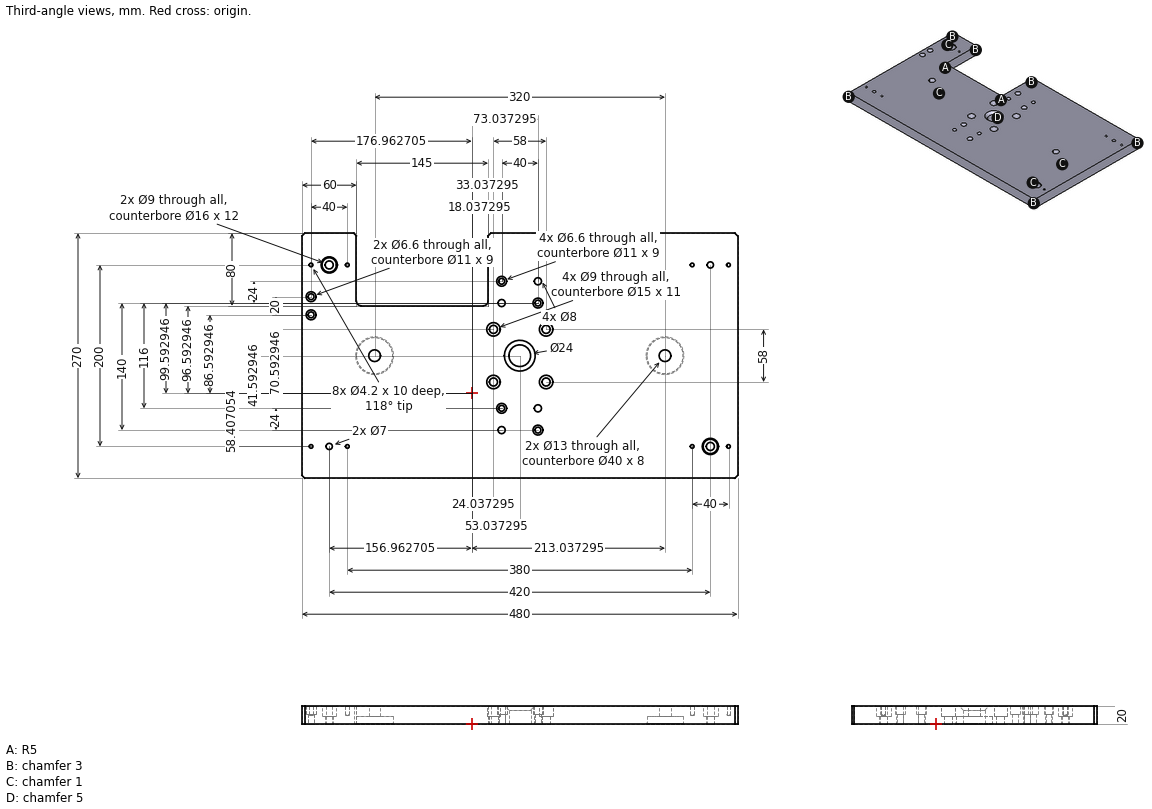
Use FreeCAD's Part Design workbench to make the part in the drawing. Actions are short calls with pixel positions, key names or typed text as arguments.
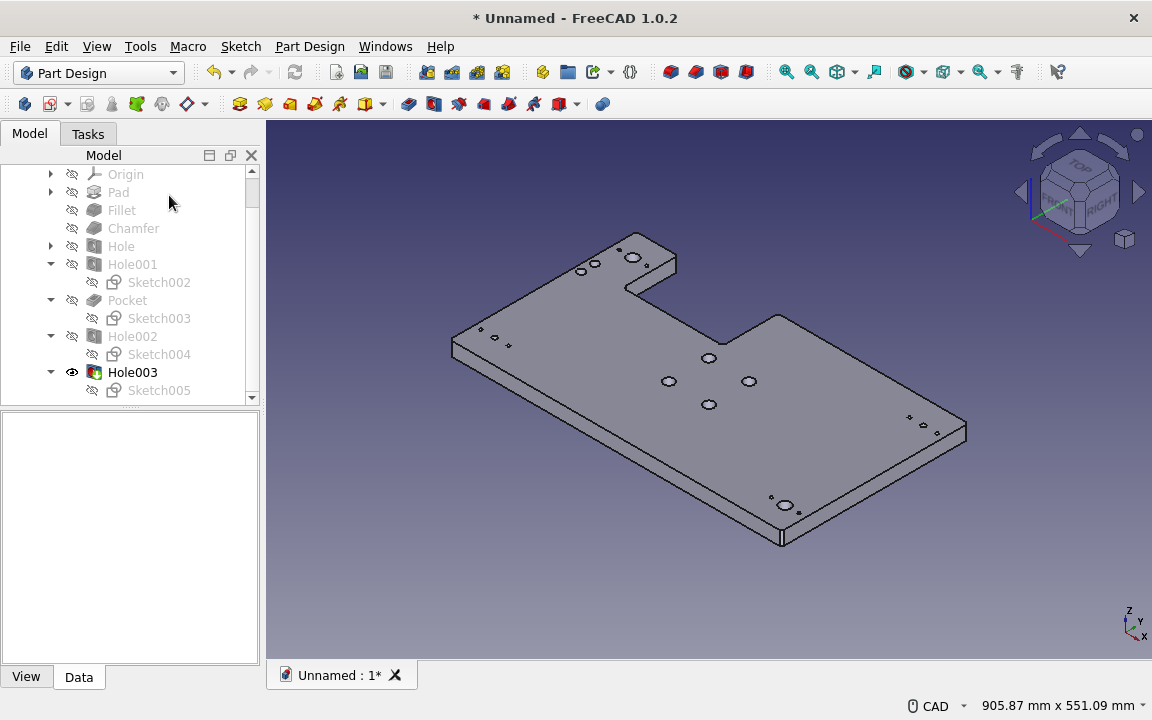
click(804, 435)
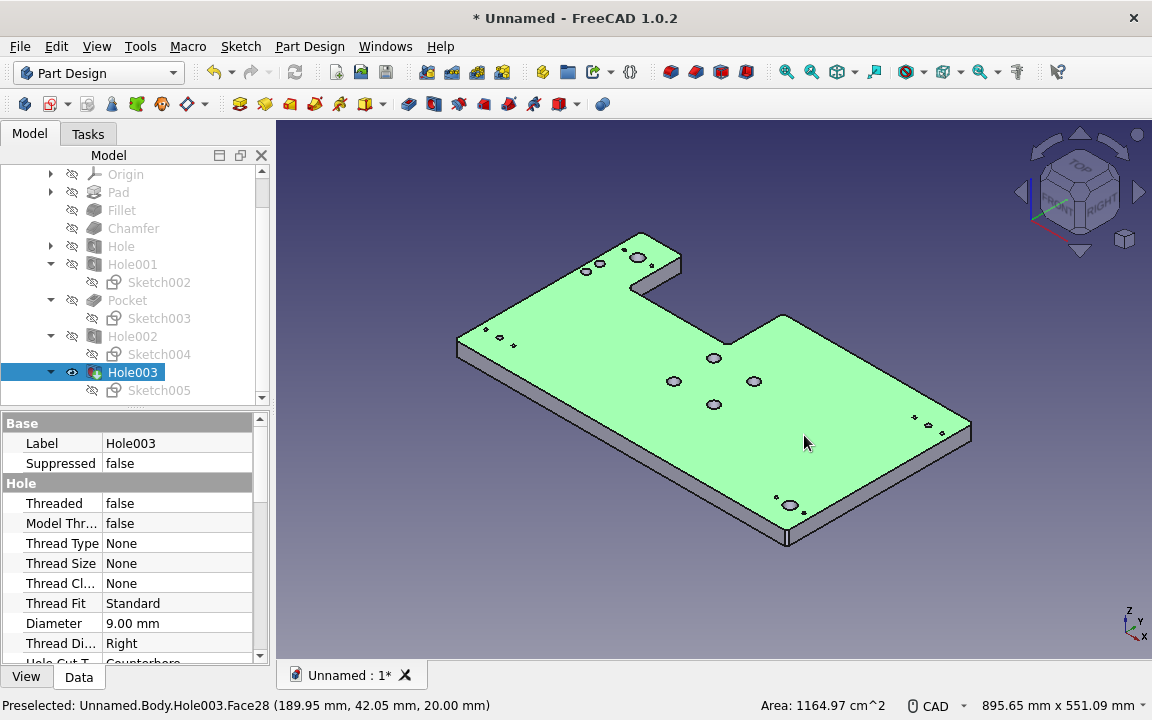
click(50, 104)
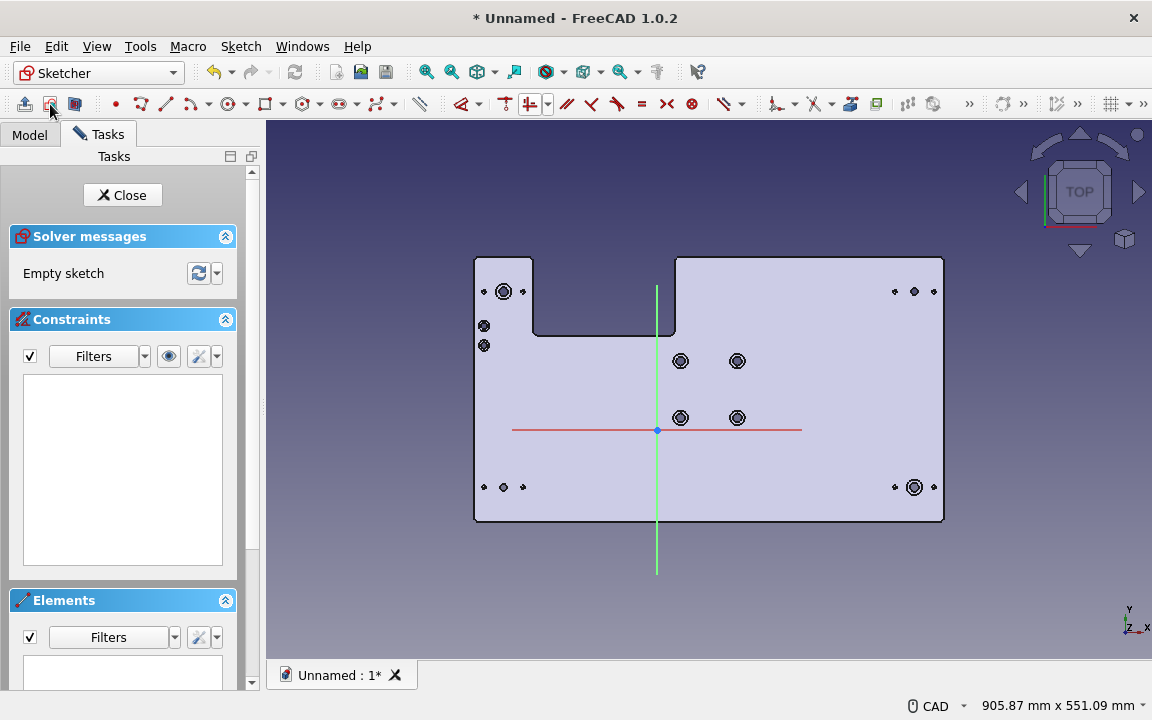
scroll(738, 390, up, 4)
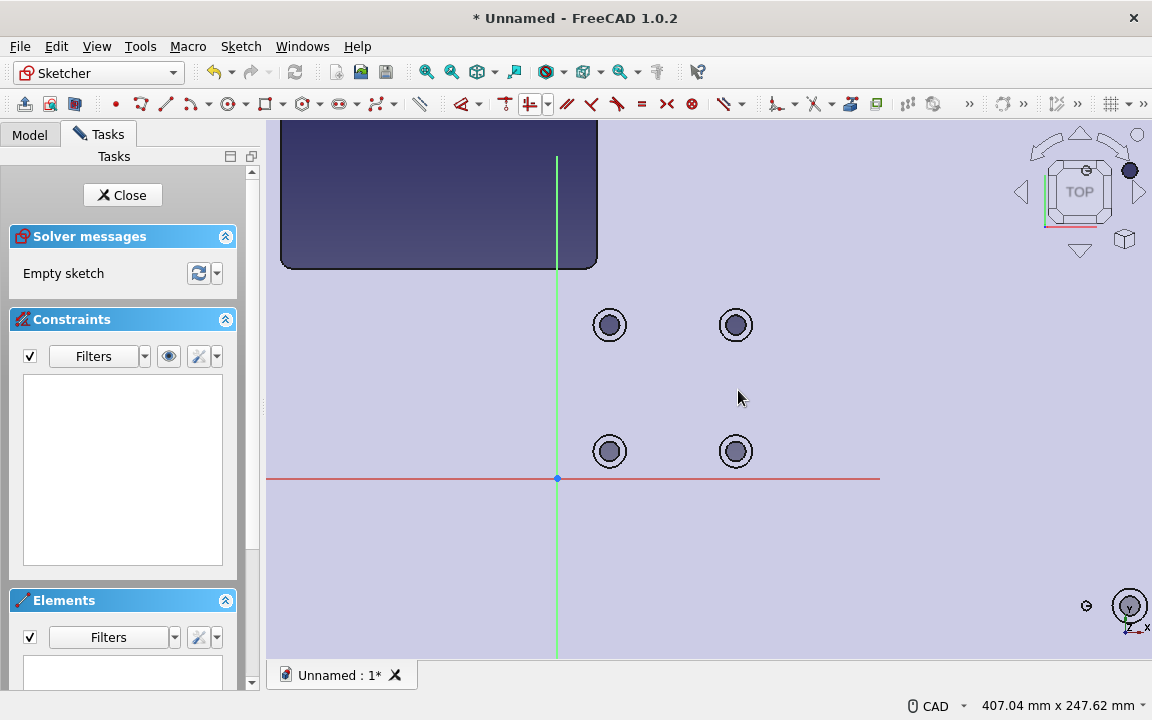
key(g)
key(c)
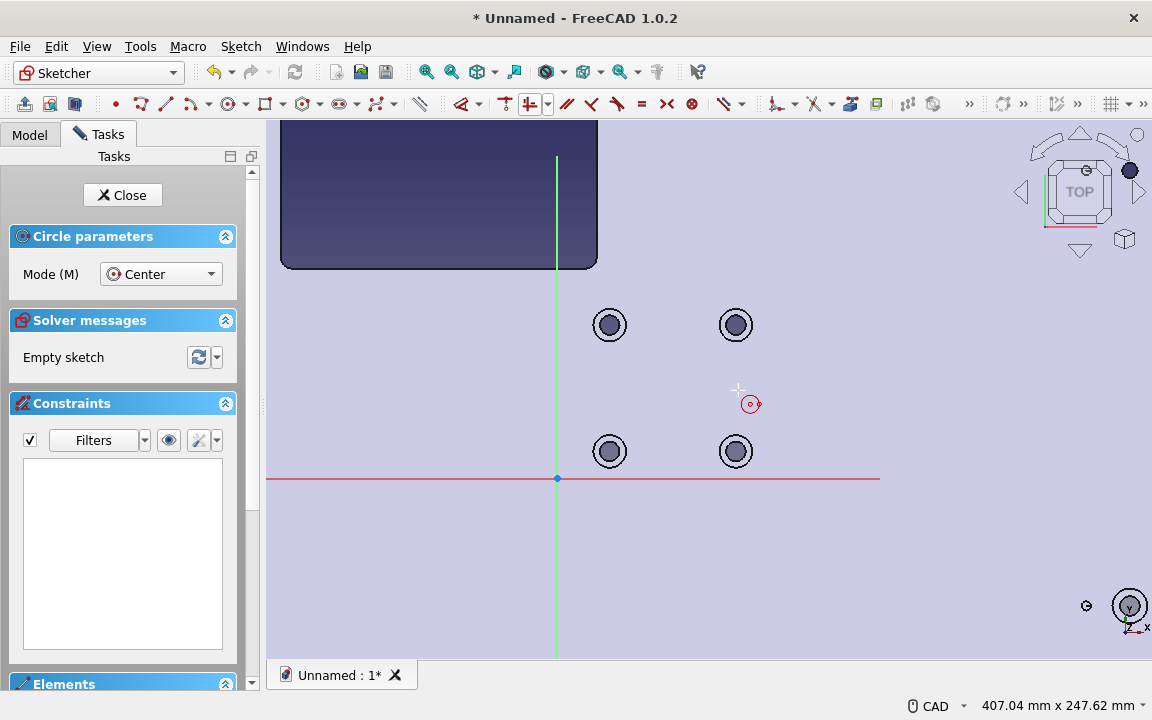
scroll(629, 210, up, 6)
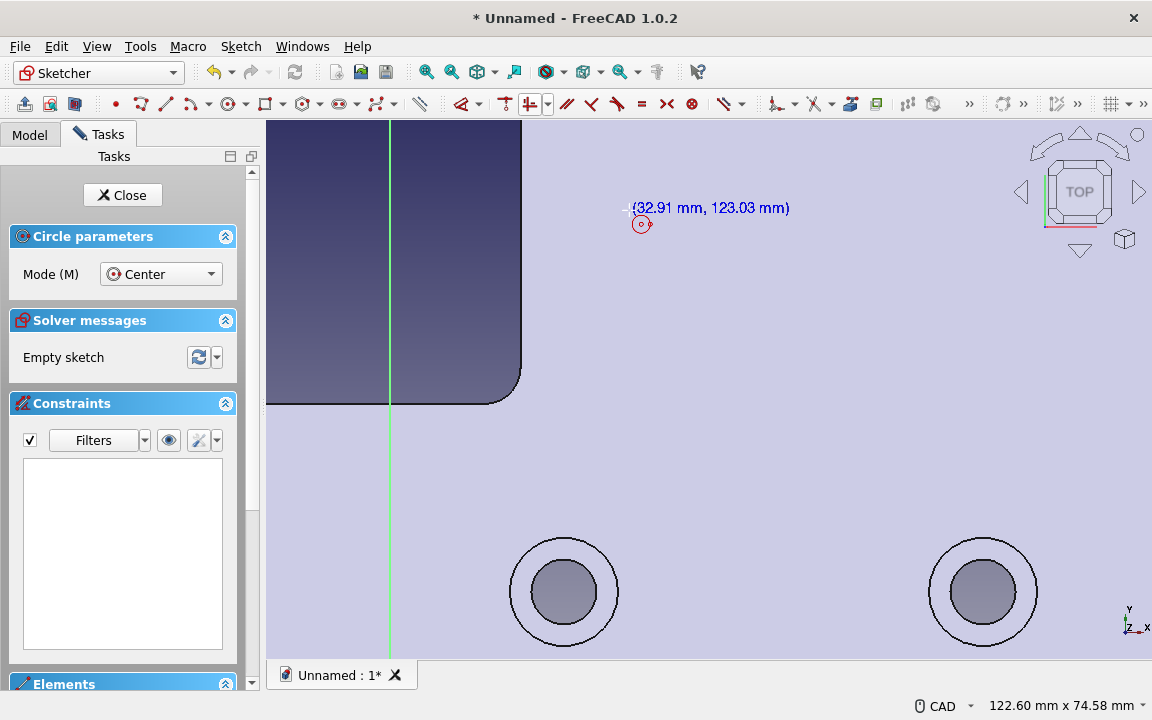
click(629, 209)
click(646, 192)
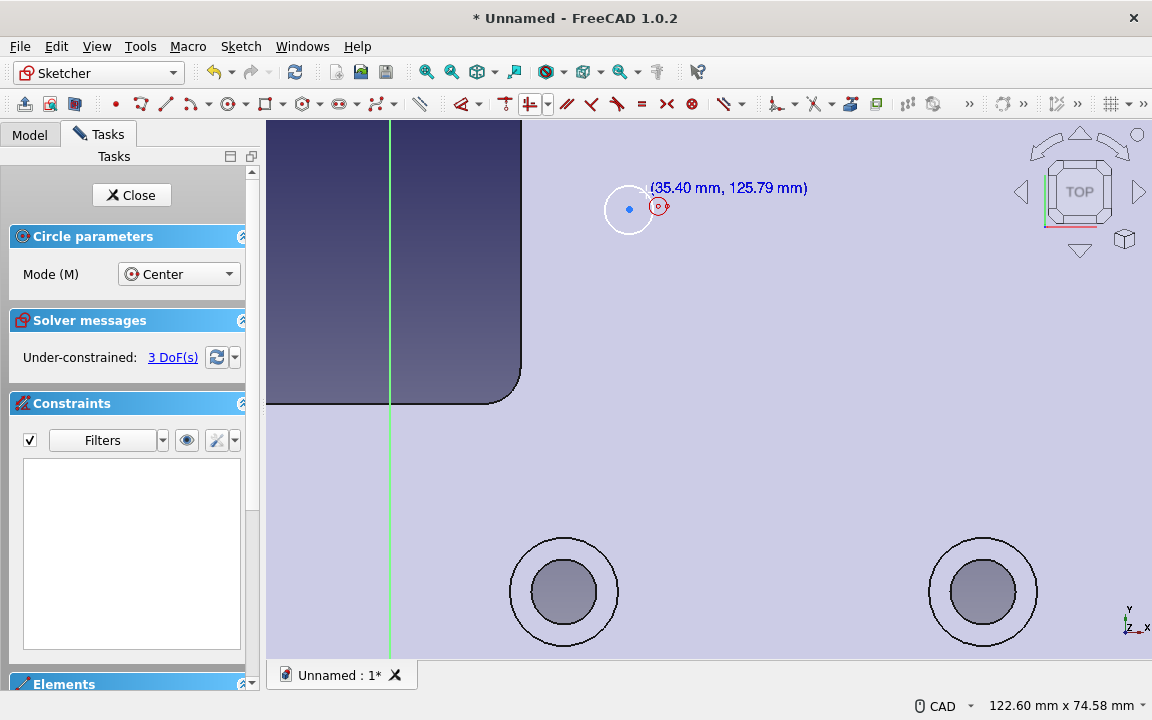
click(918, 382)
click(935, 365)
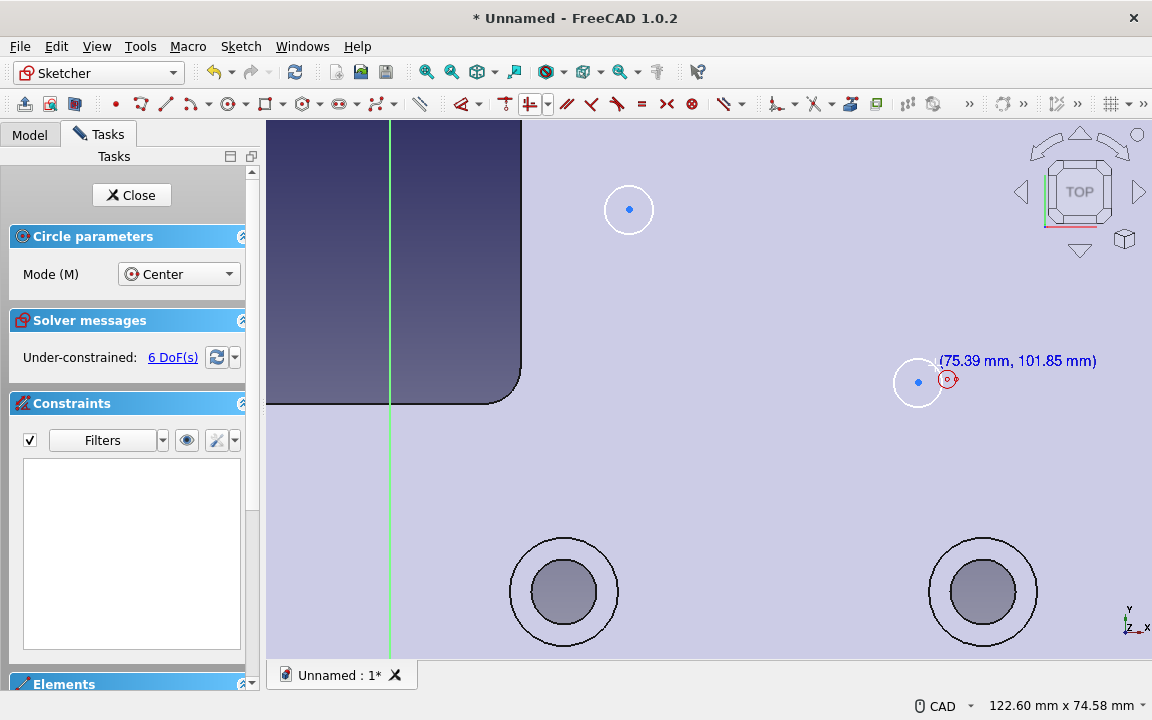
scroll(629, 212, down, 6)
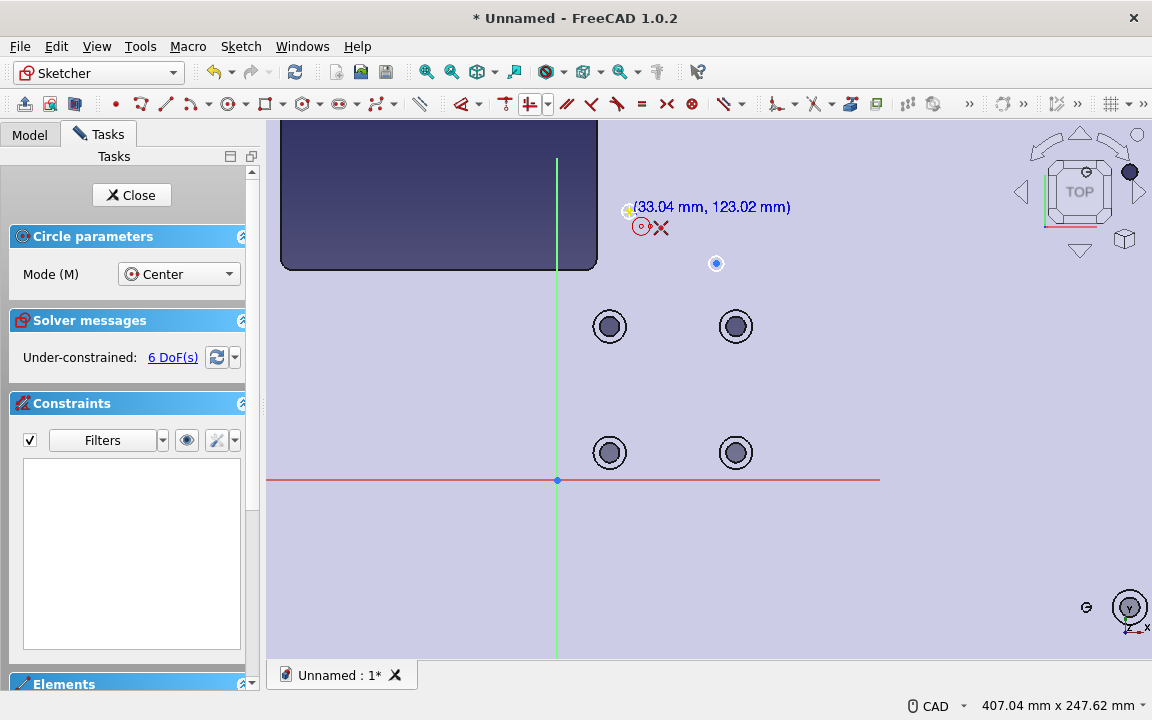
scroll(629, 516, up, 6)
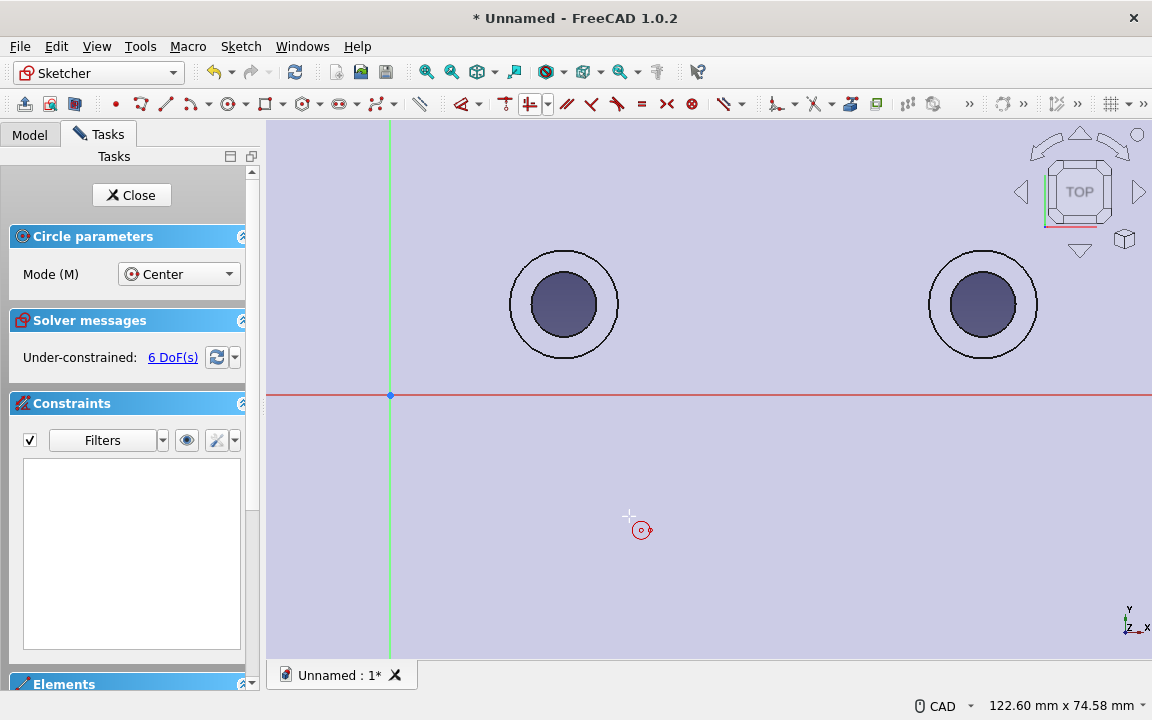
click(629, 514)
click(646, 497)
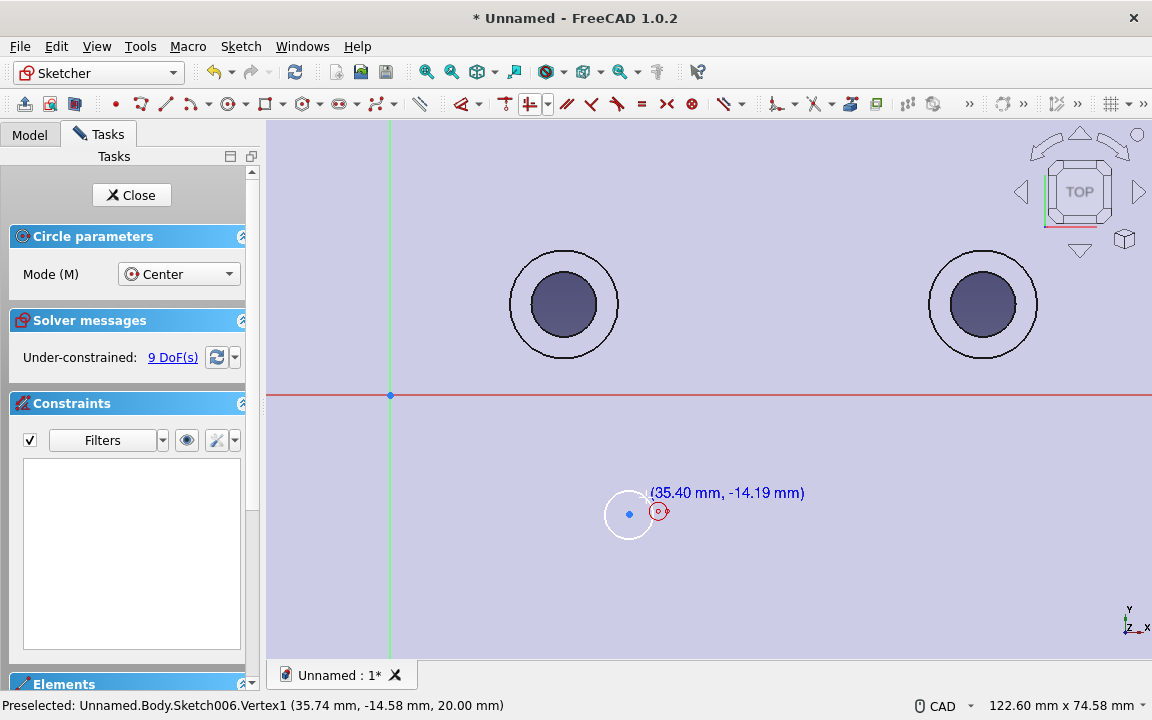
scroll(629, 516, down, 6)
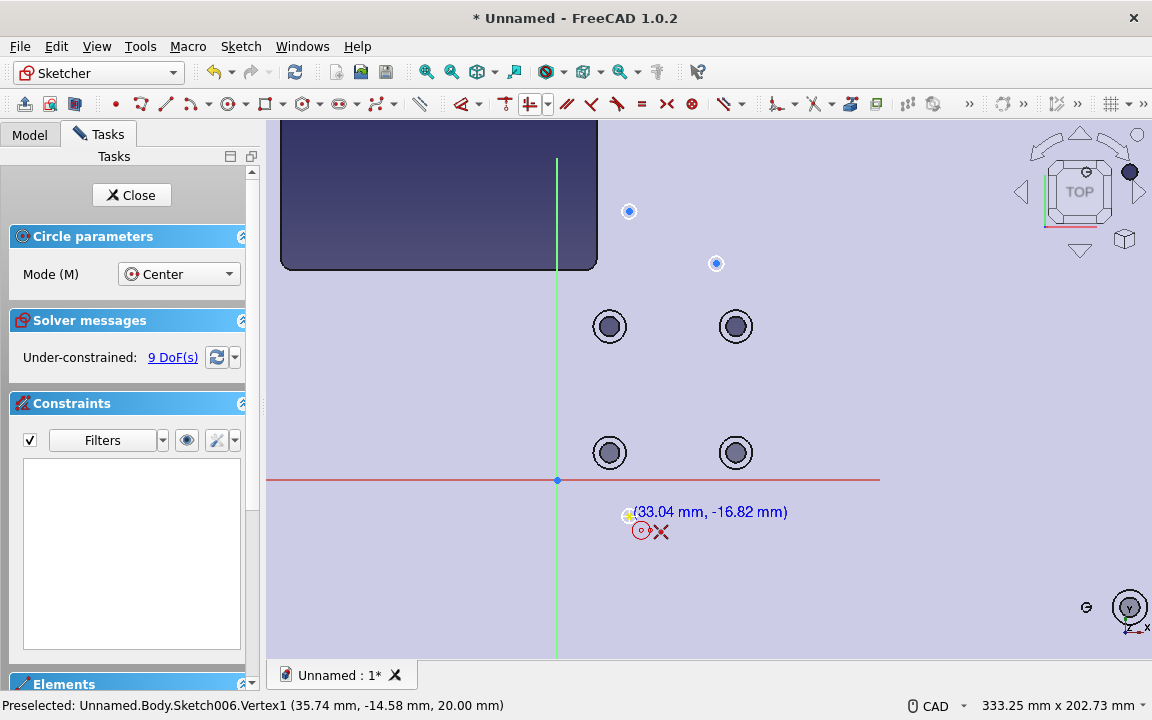
scroll(716, 568, up, 6)